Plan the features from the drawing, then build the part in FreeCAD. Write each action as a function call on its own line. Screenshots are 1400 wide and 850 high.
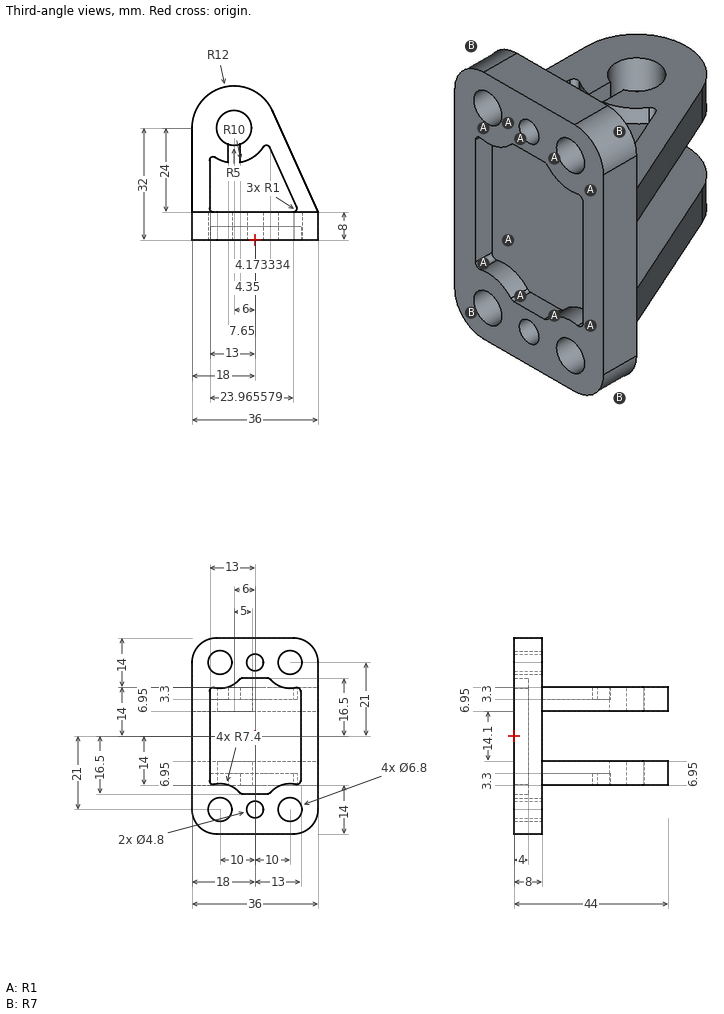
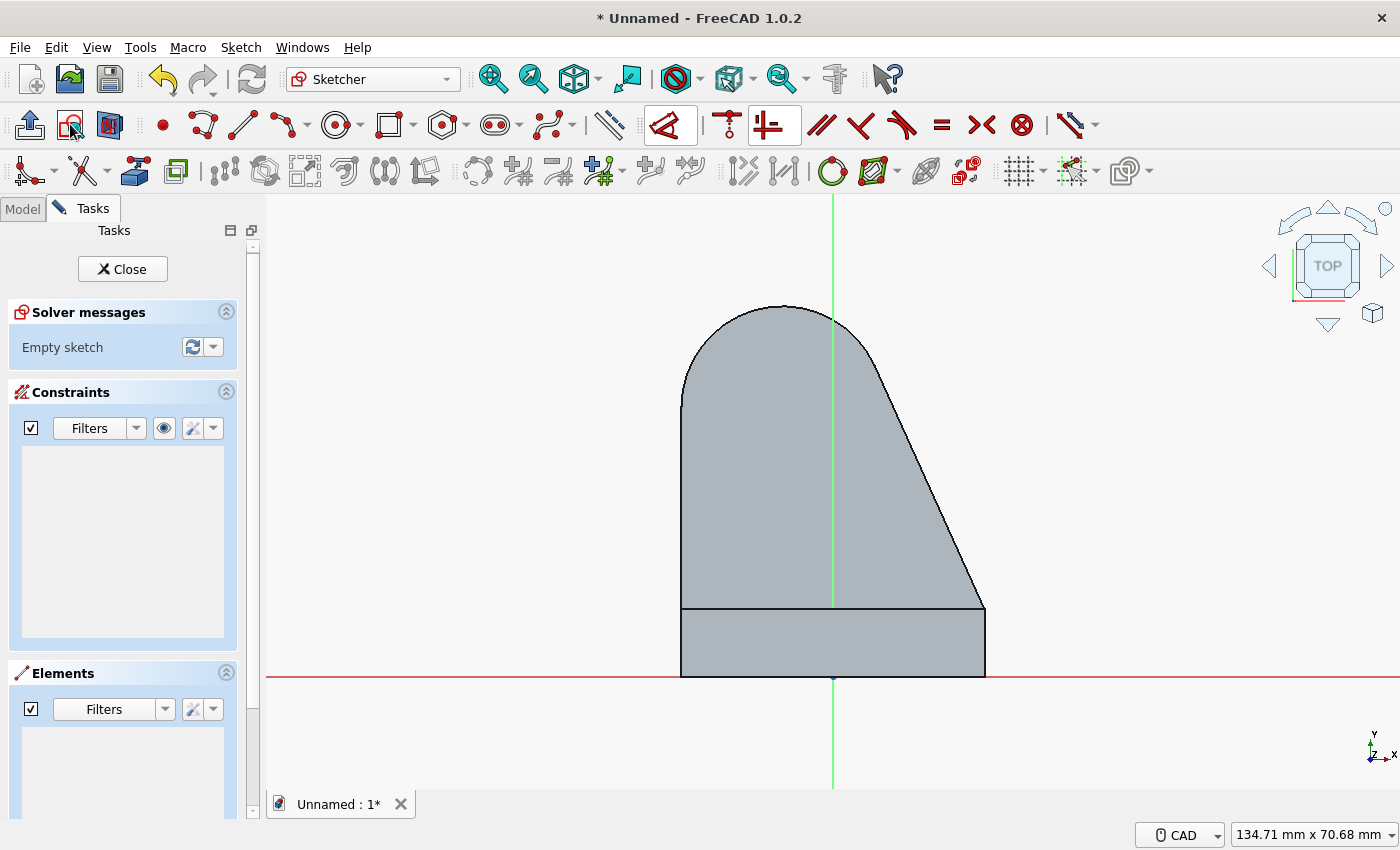
key(q)
key(s)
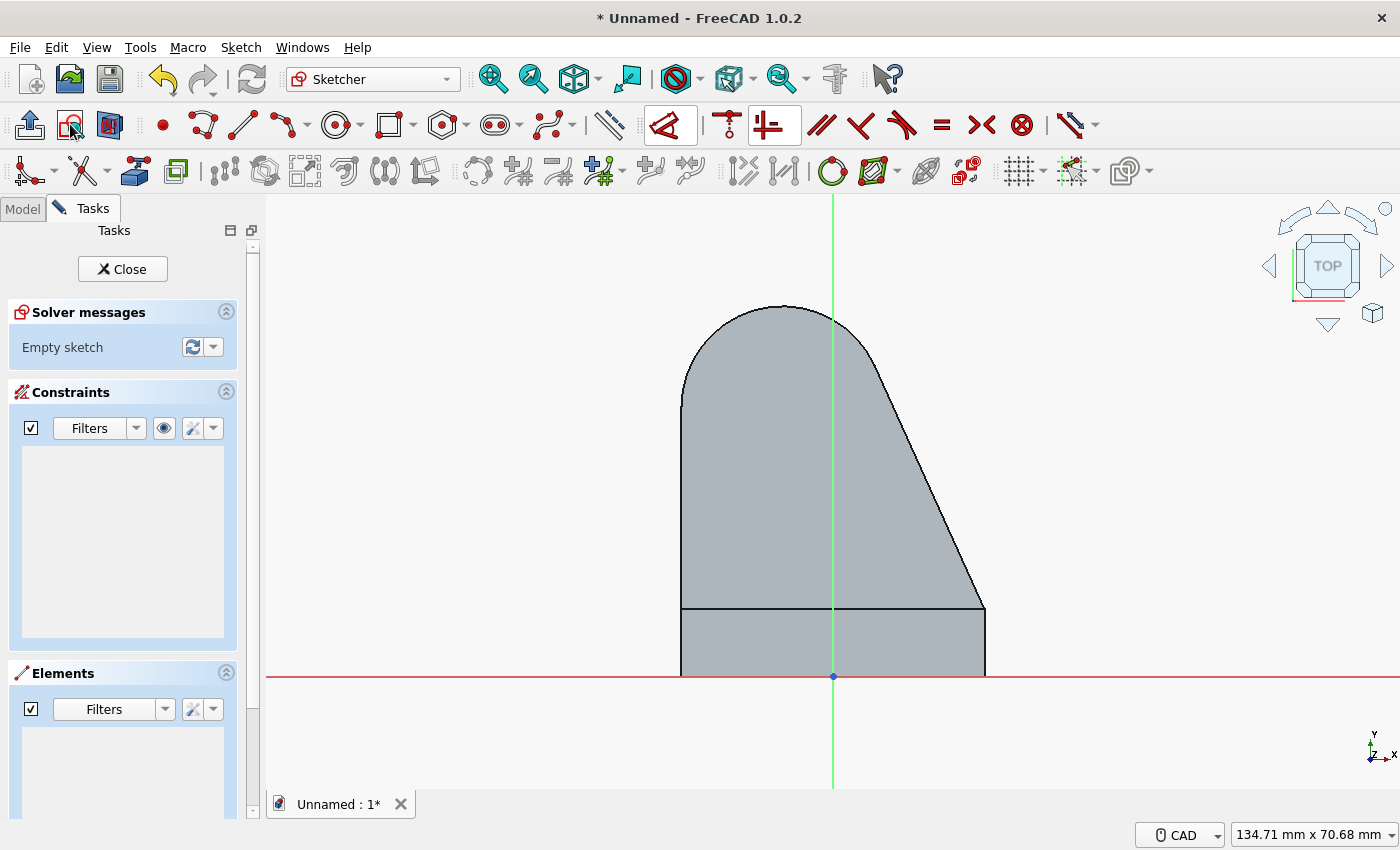
scroll(906, 649, up, 3)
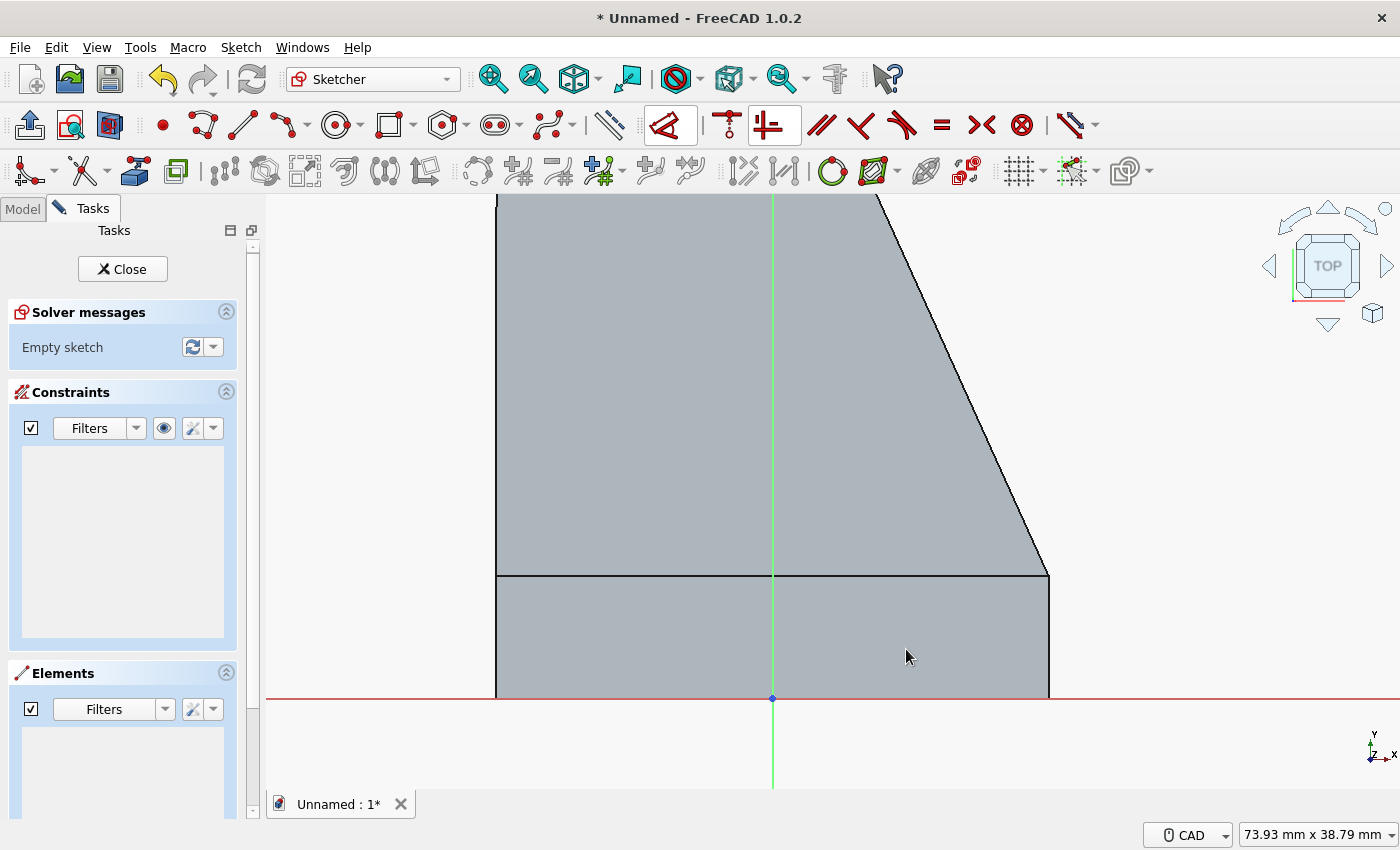
key(g)
key(m)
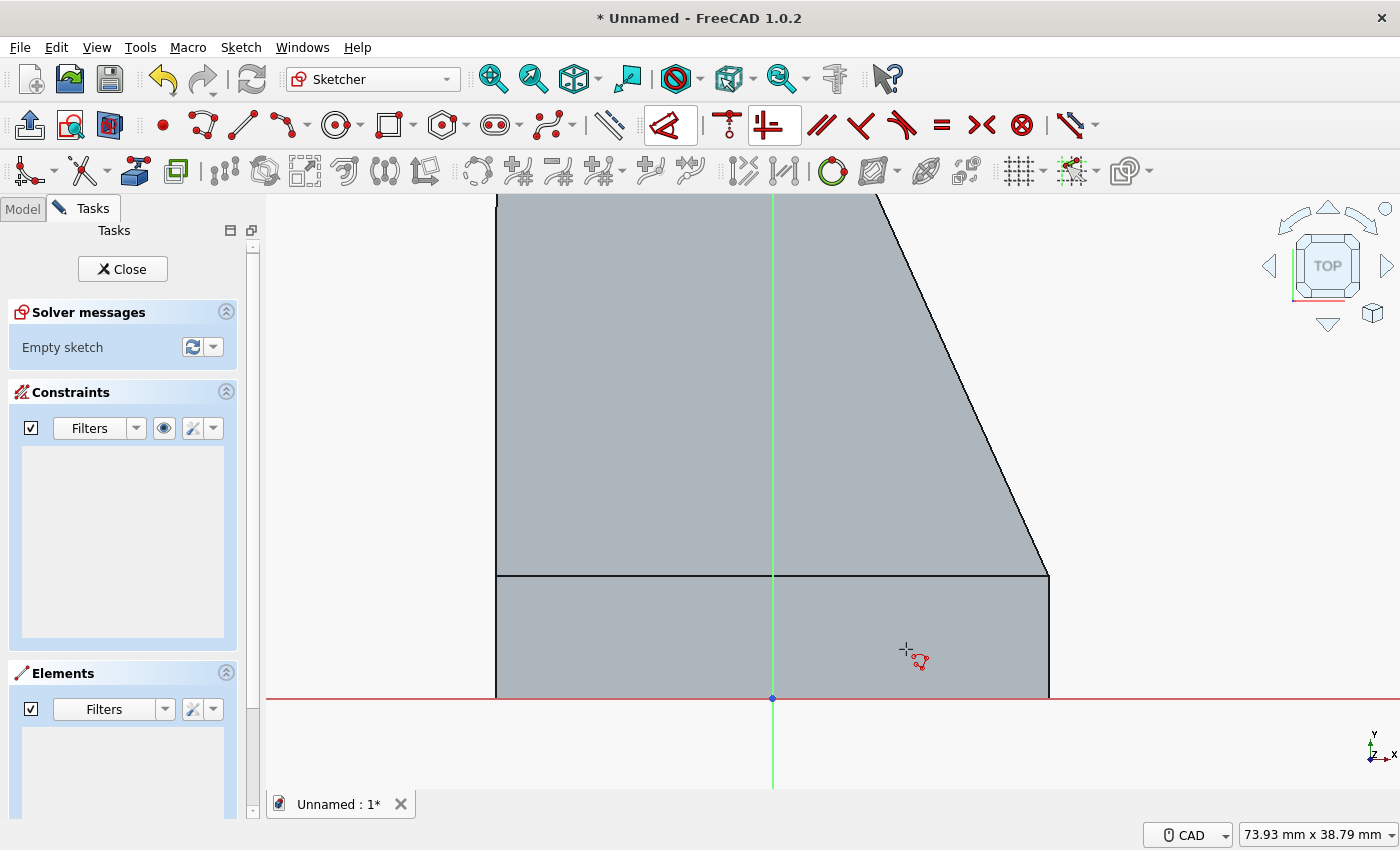
click(573, 349)
click(573, 576)
click(941, 576)
right_click(941, 576)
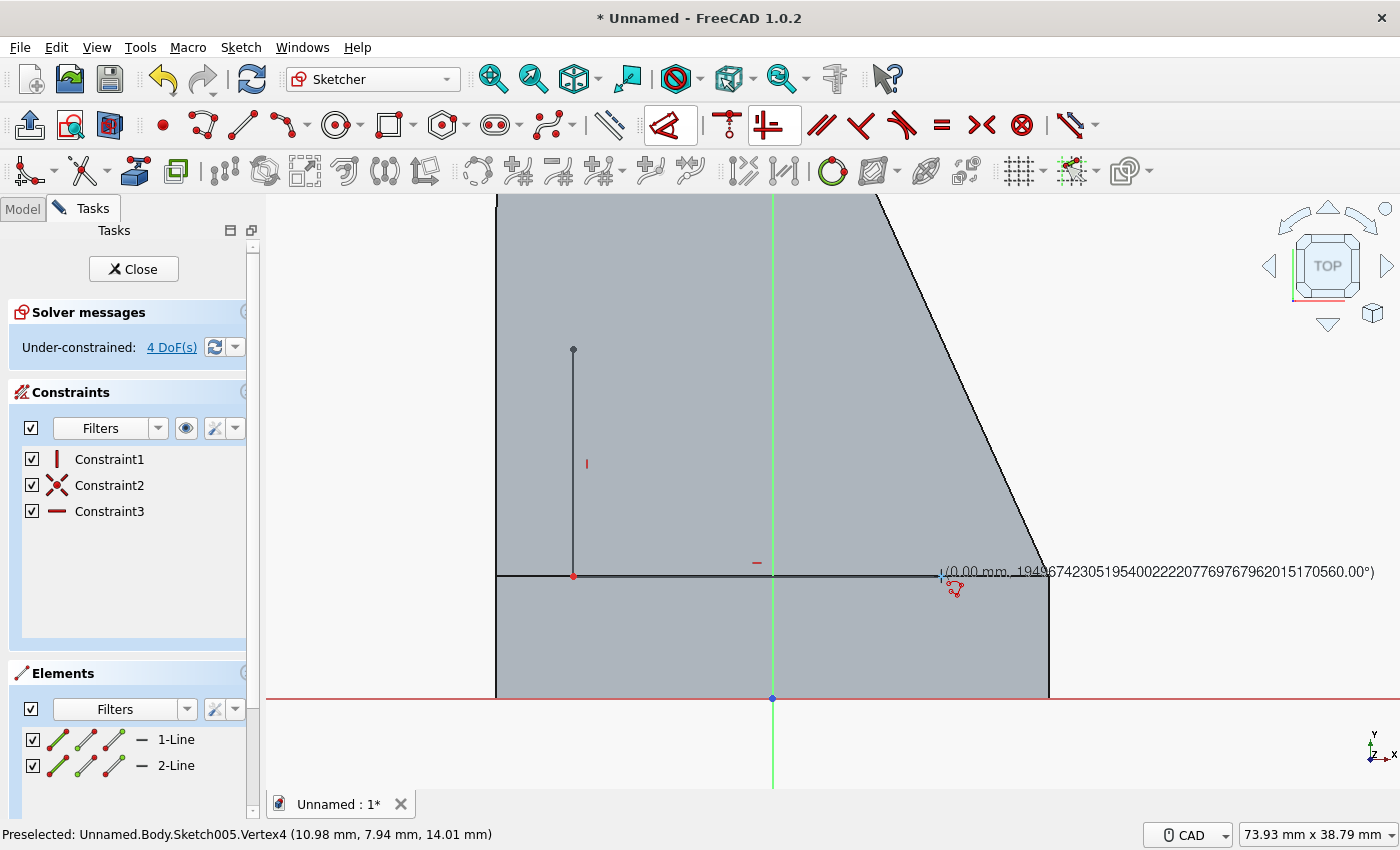
key(g)
key(l)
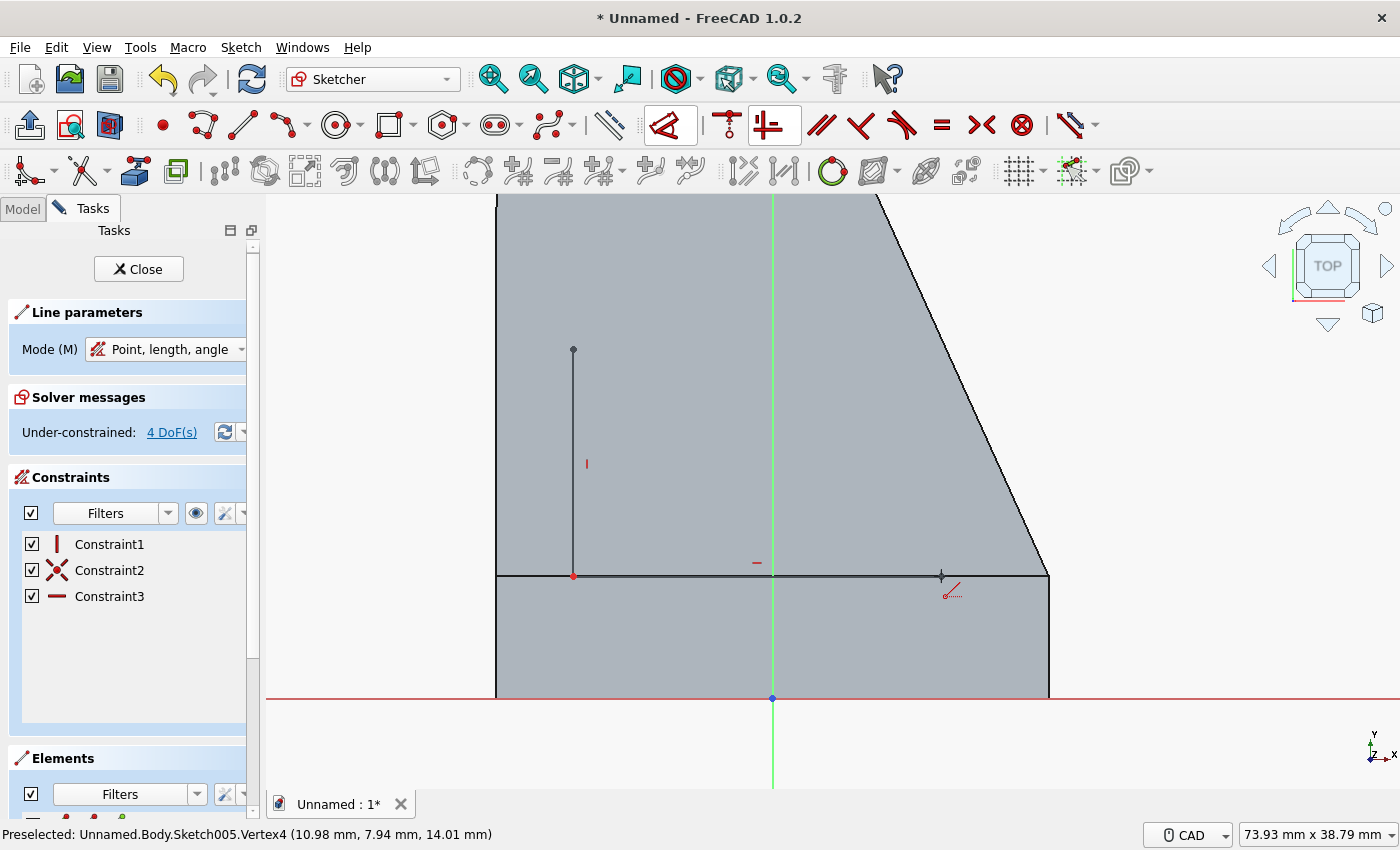
click(955, 554)
click(837, 293)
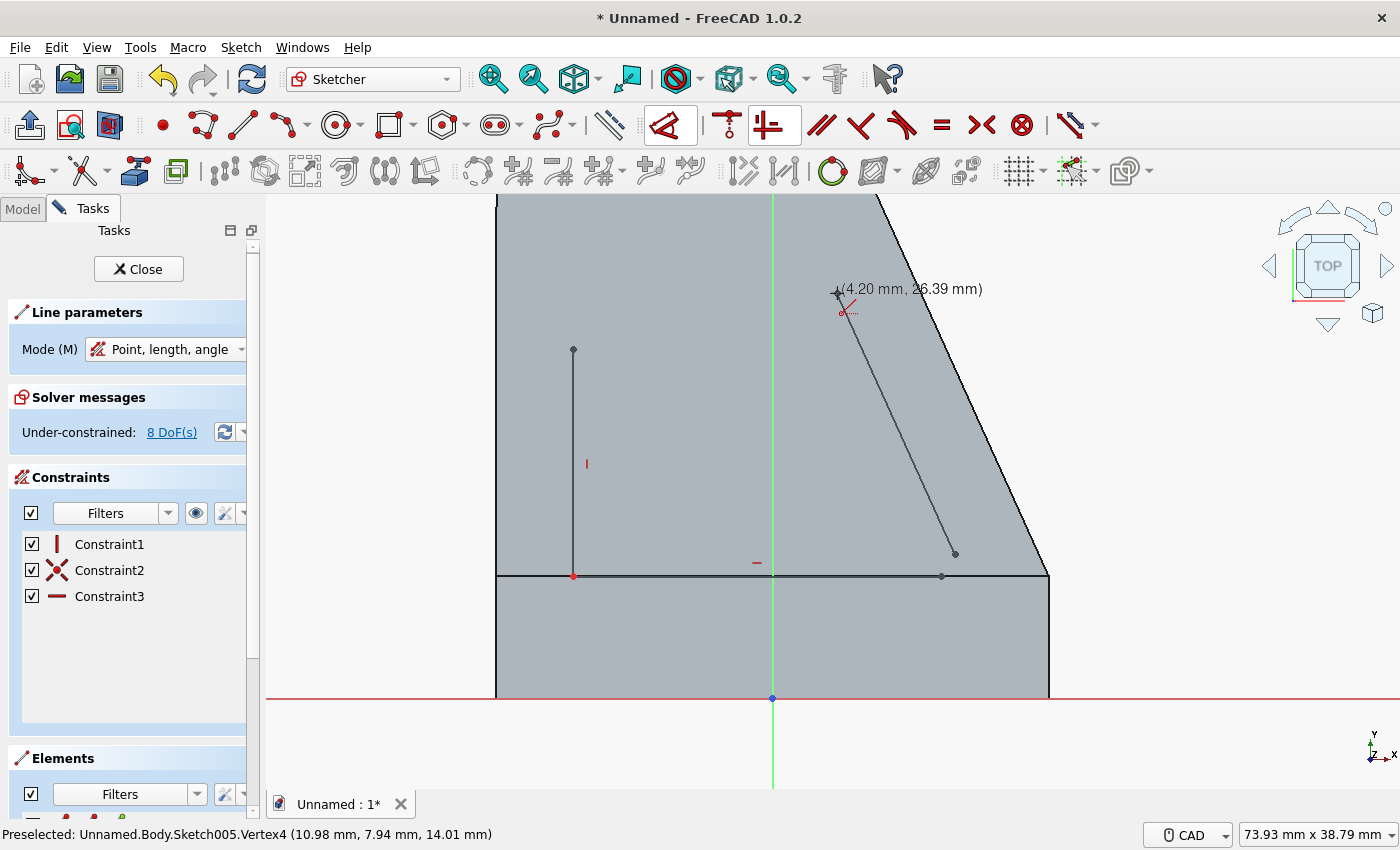
click(284, 126)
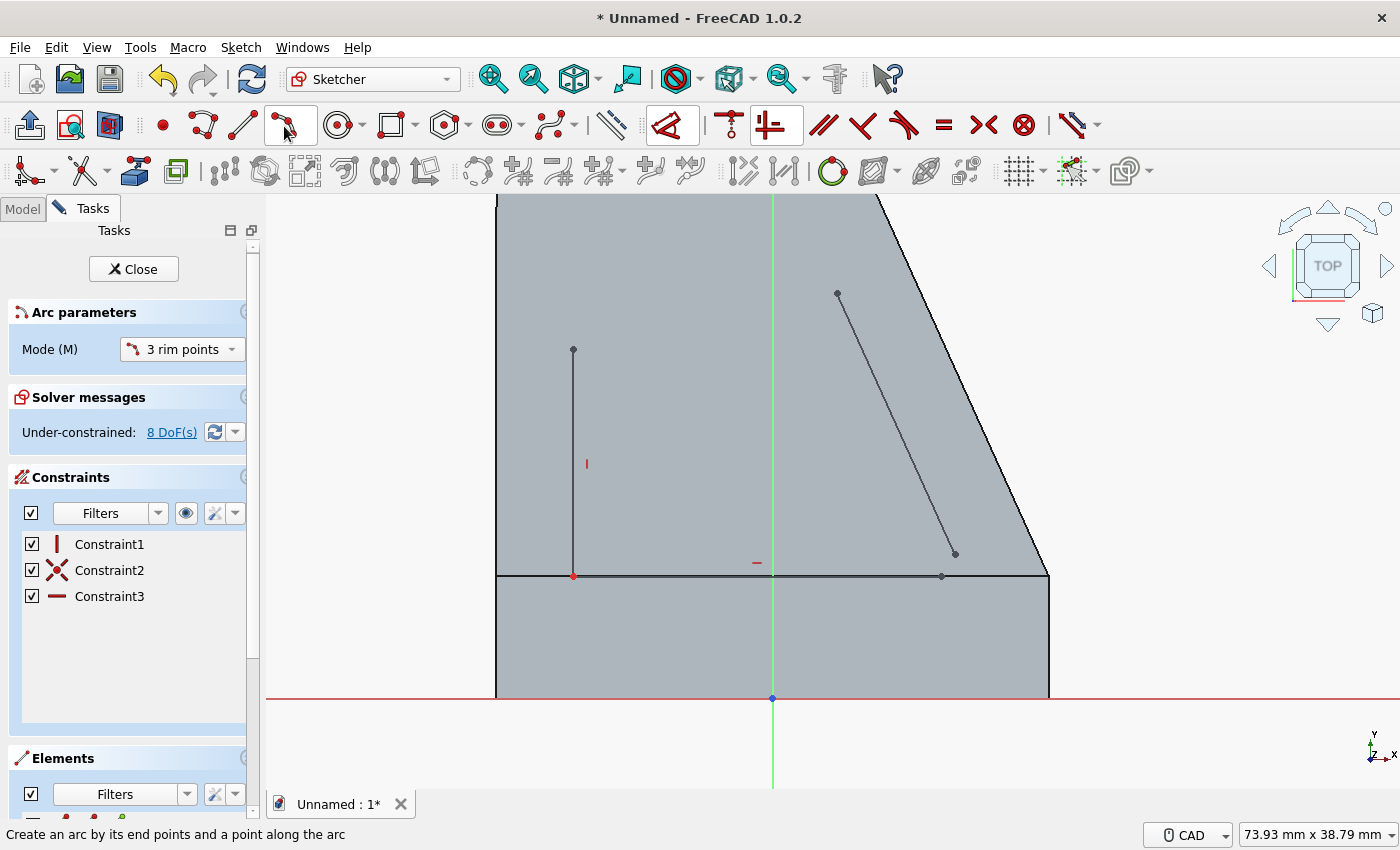
click(941, 577)
click(955, 555)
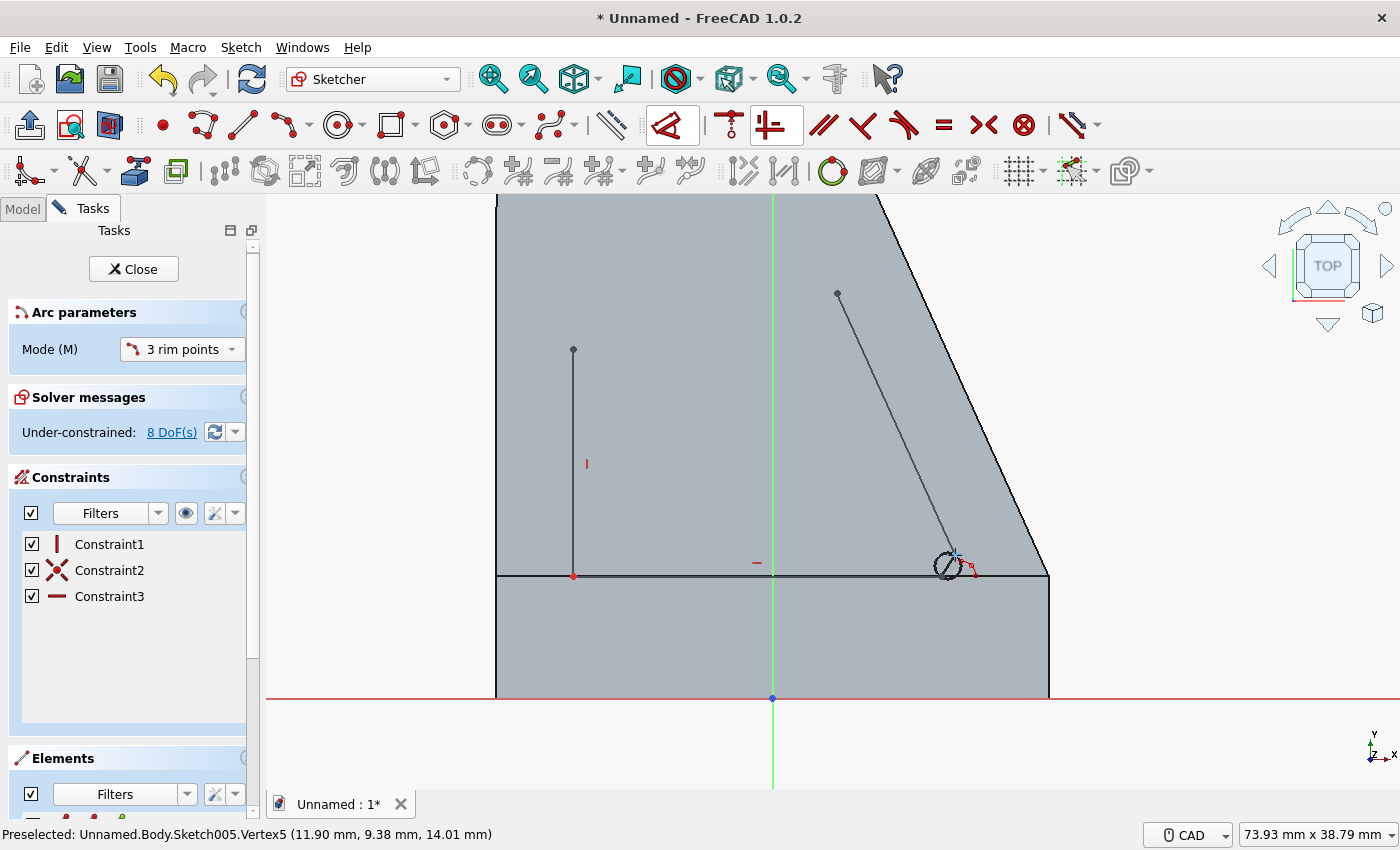
scroll(954, 569, up, 5)